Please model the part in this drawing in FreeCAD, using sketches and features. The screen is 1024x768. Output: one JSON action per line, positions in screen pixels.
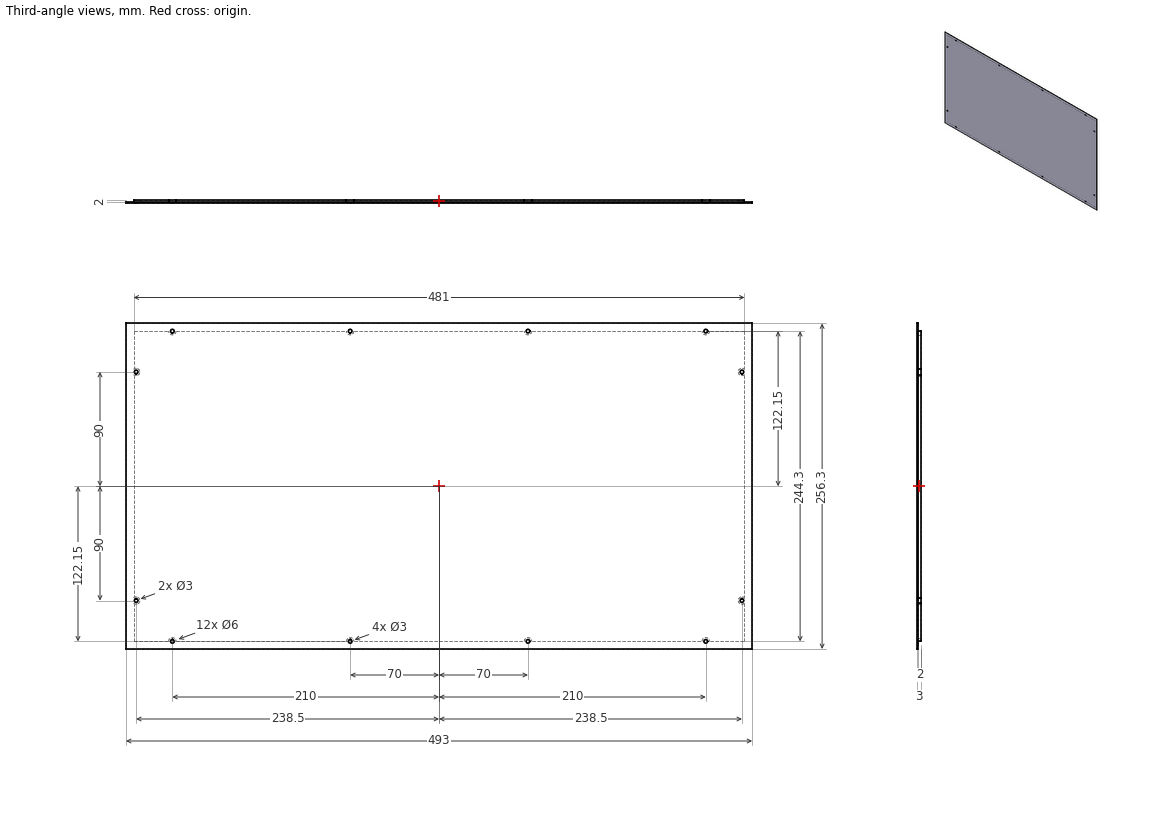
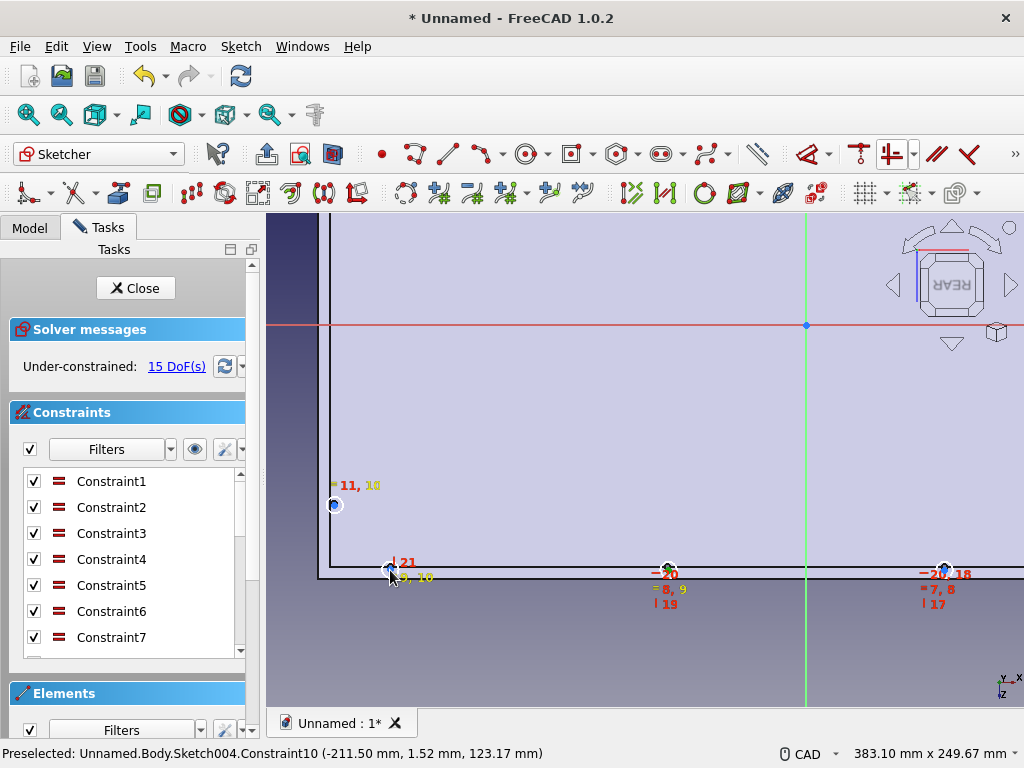
{"action": "scroll", "coordinate": [390, 570], "scroll_direction": "up", "scroll_amount": 4}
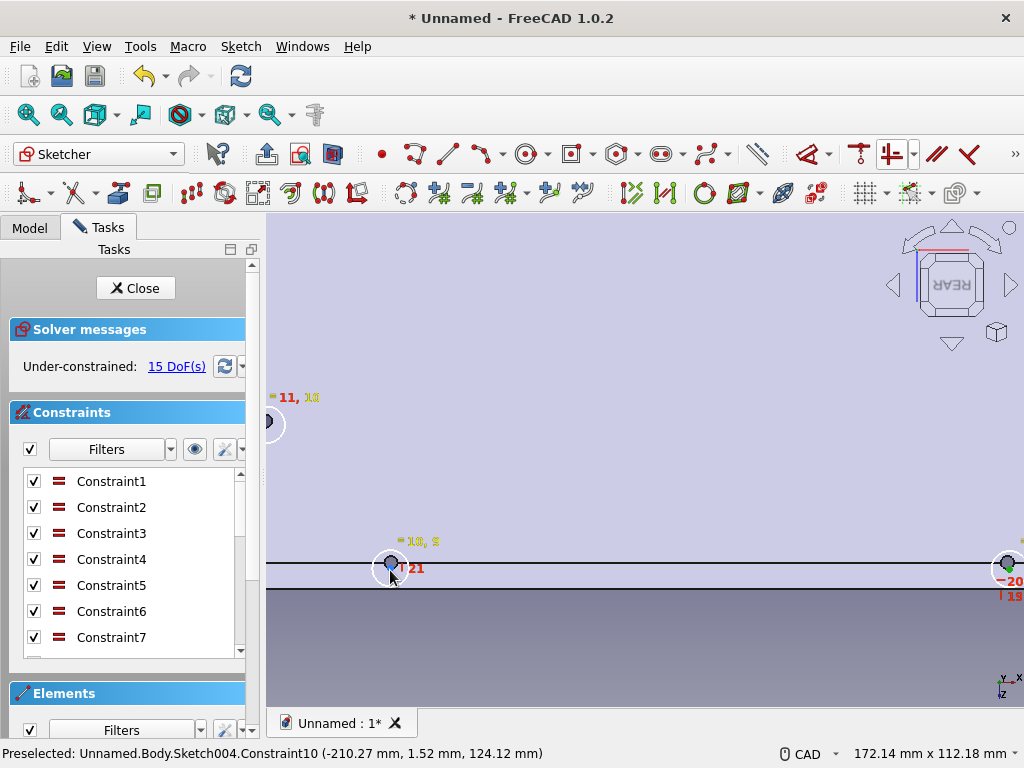
{"action": "left_click", "coordinate": [391, 568]}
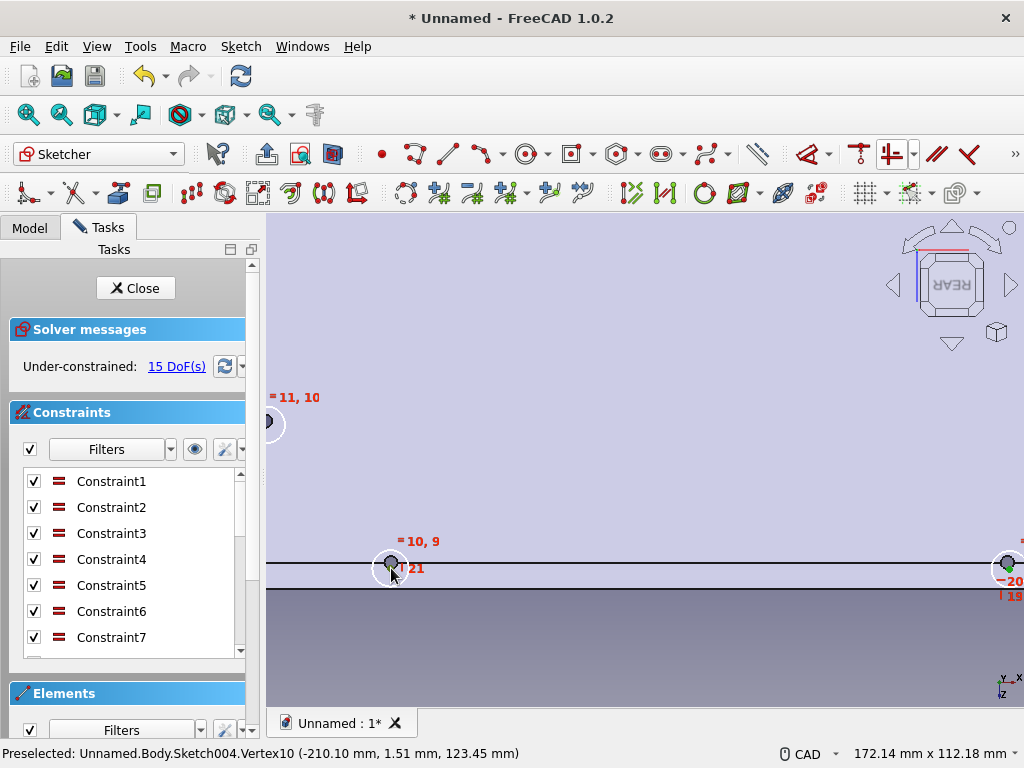
{"action": "left_click", "coordinate": [914, 154]}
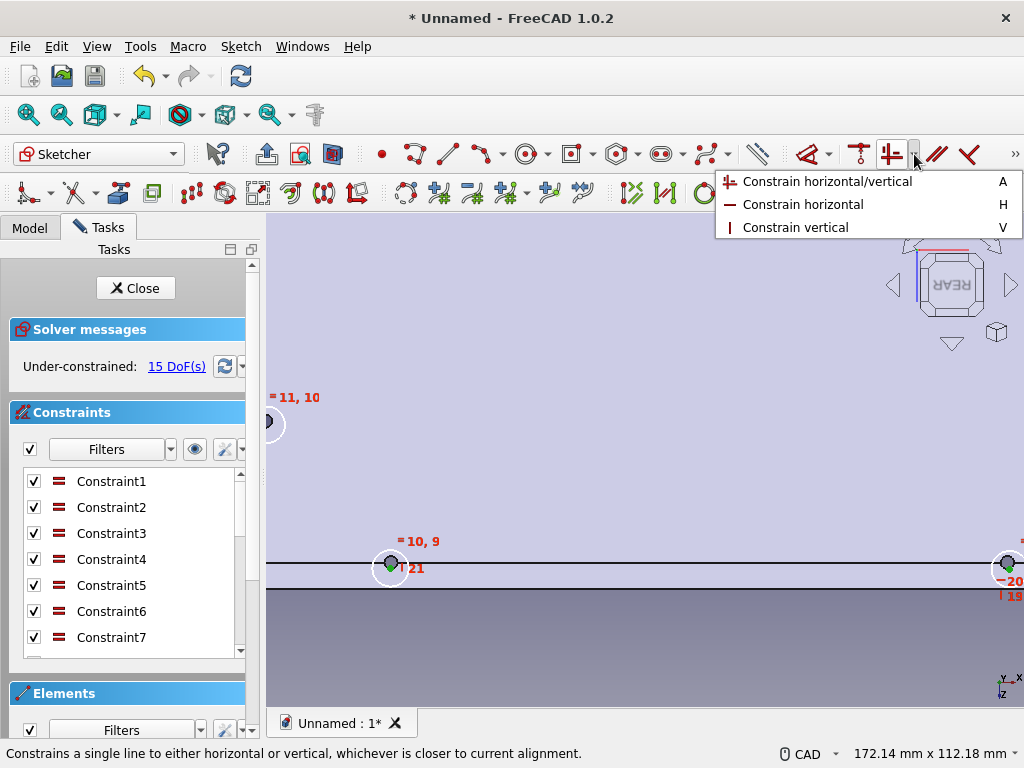
{"action": "left_click", "coordinate": [869, 204]}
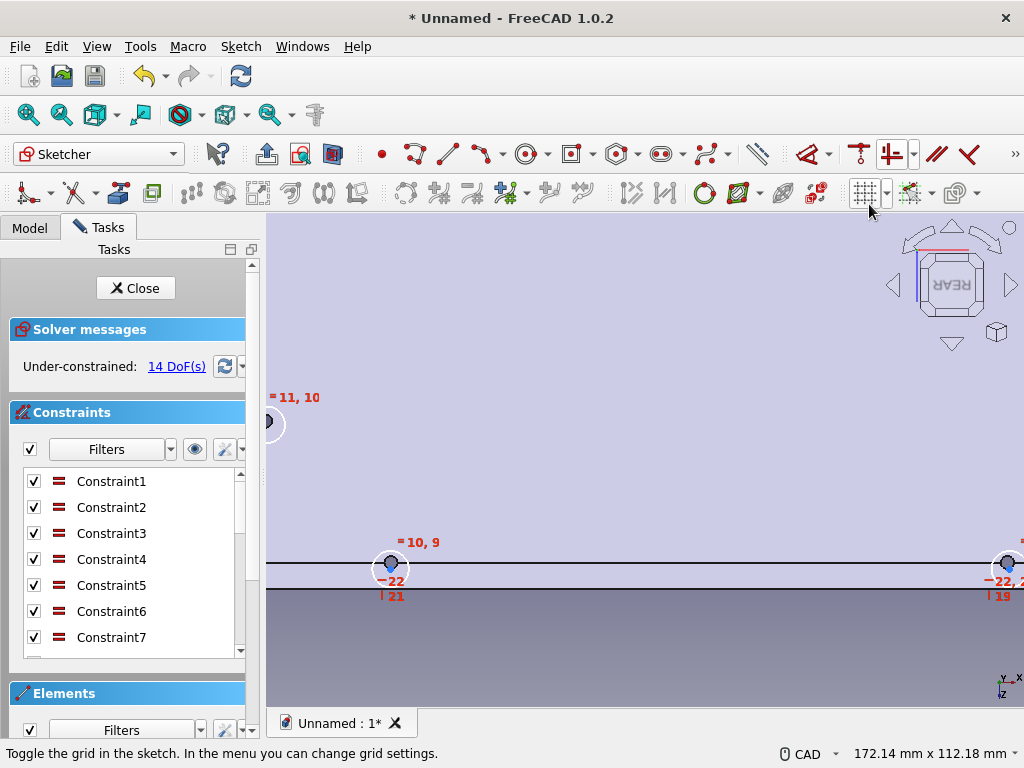
{"action": "scroll", "coordinate": [389, 570], "scroll_direction": "down", "scroll_amount": 8}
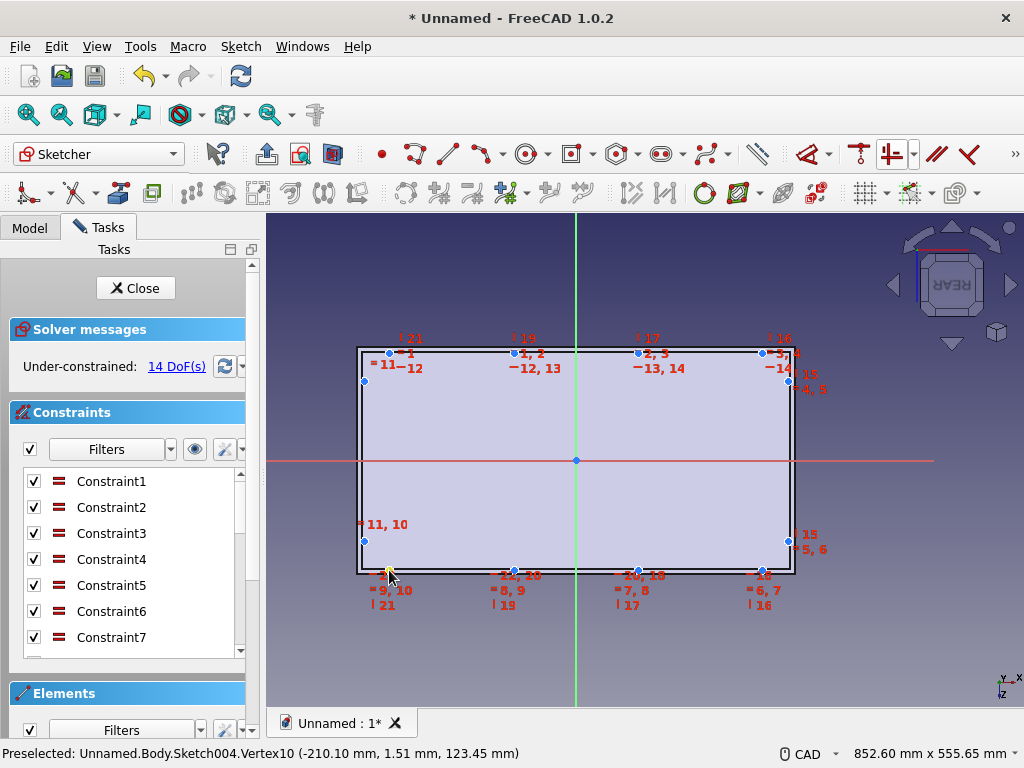
{"action": "left_click", "coordinate": [364, 541]}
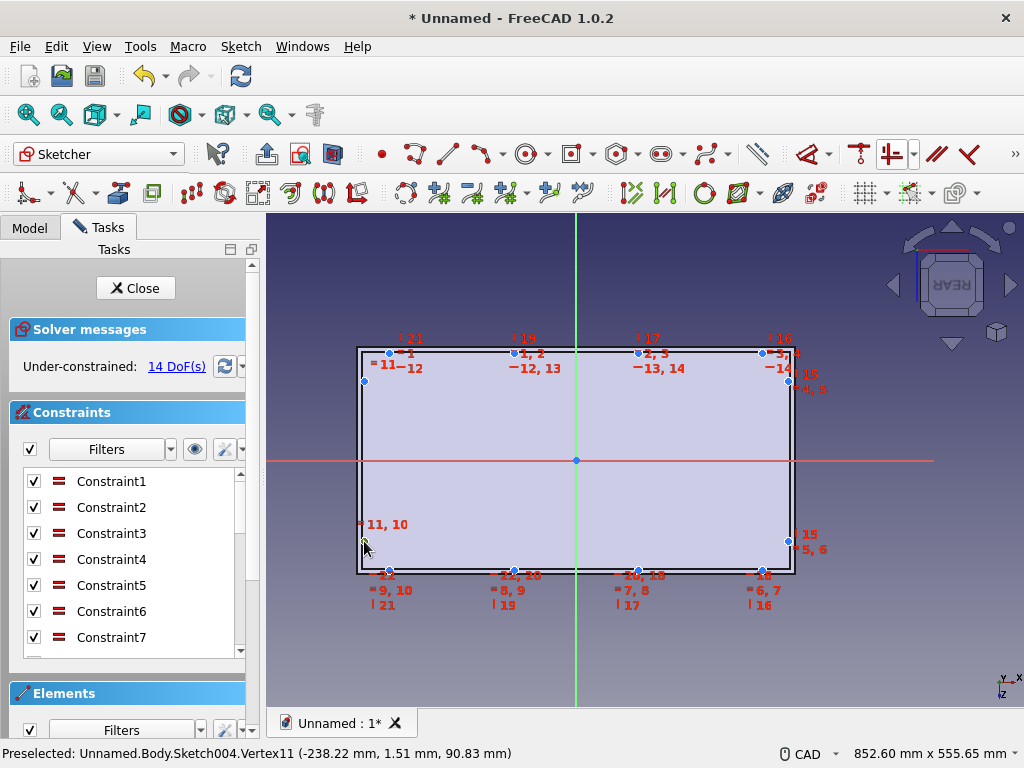
{"action": "left_click", "coordinate": [364, 381]}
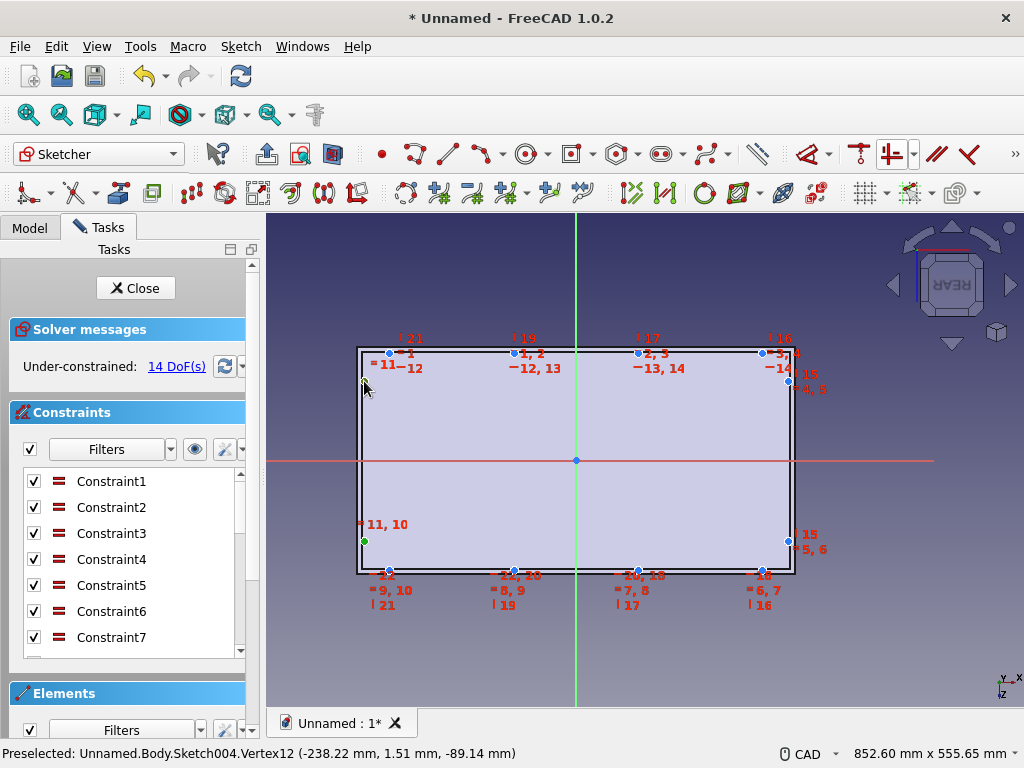
{"action": "left_click", "coordinate": [914, 154]}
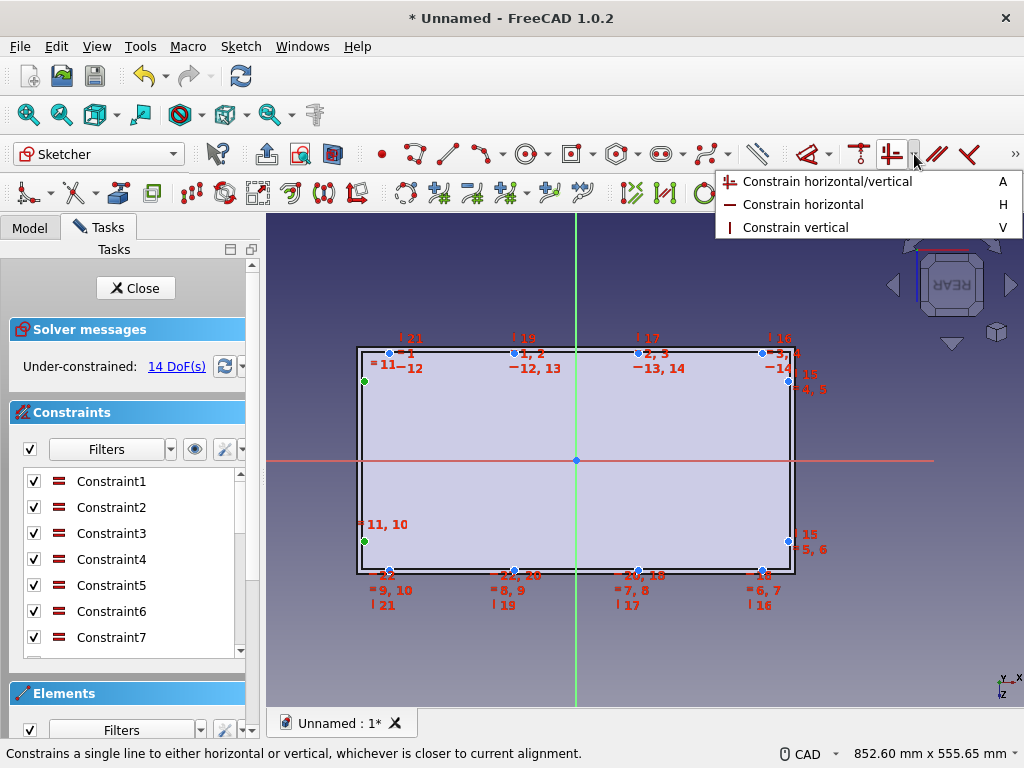
{"action": "left_click", "coordinate": [869, 228]}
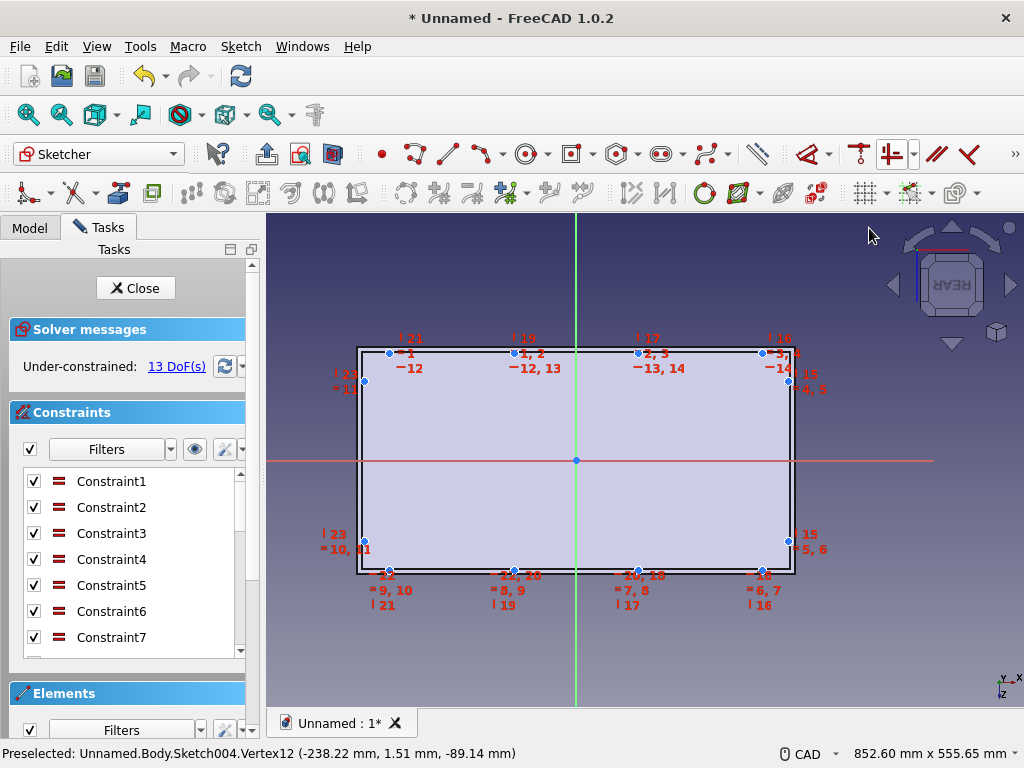
{"action": "left_click", "coordinate": [806, 154]}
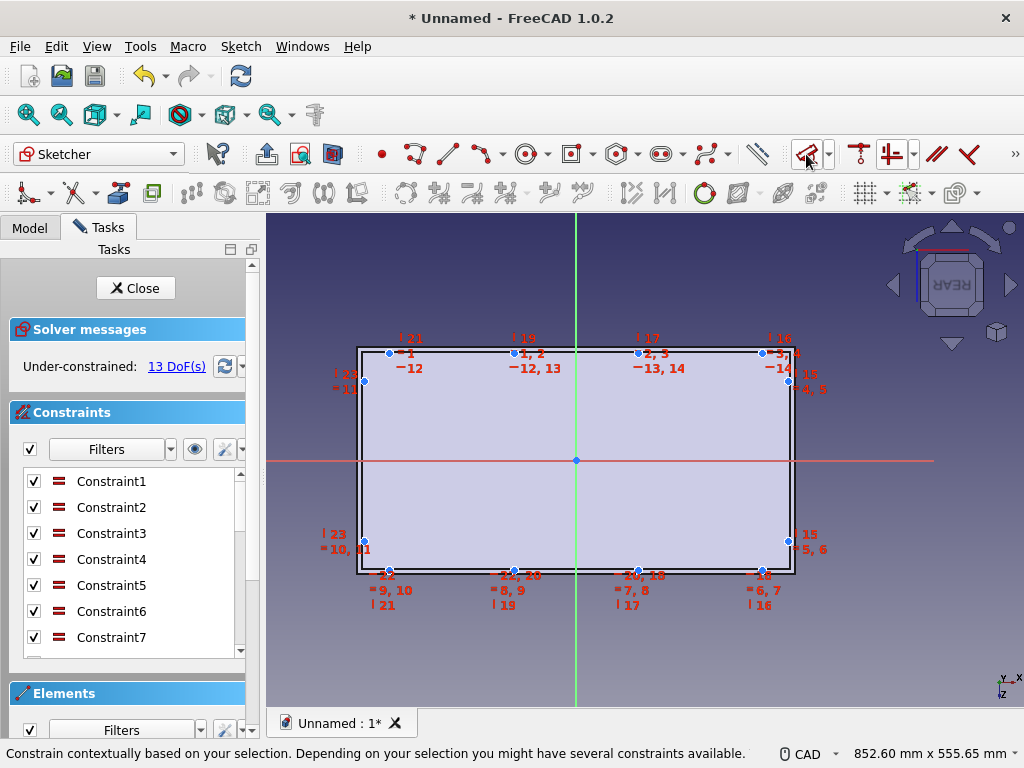
{"action": "scroll", "coordinate": [390, 350], "scroll_direction": "up", "scroll_amount": 11}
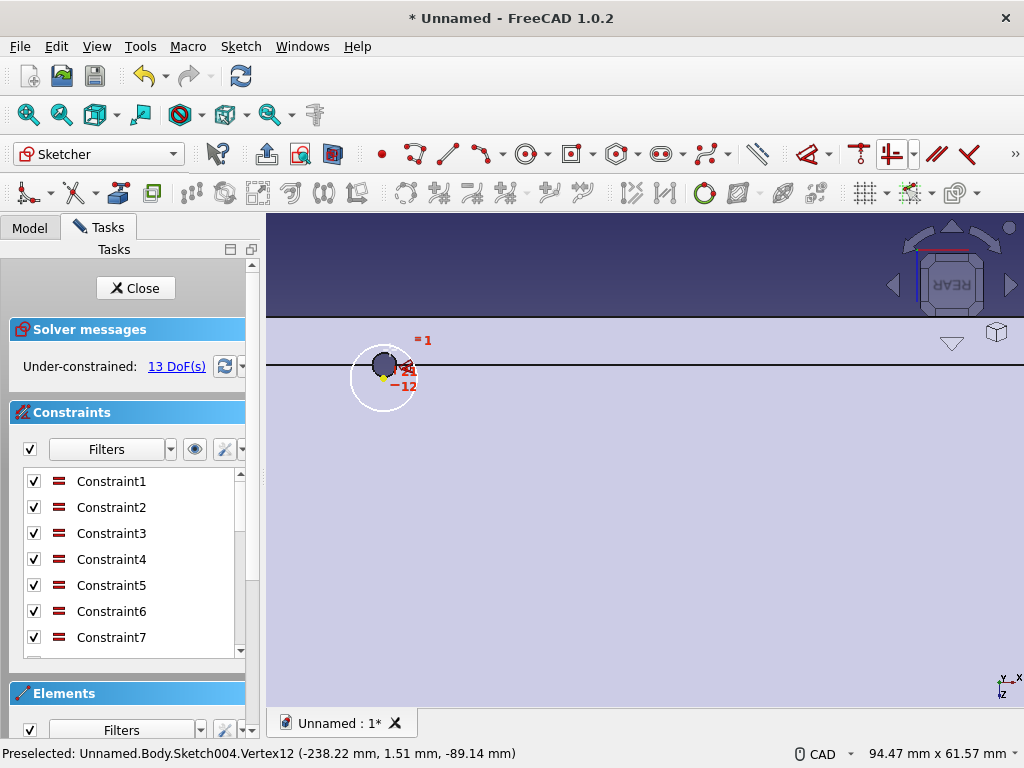
{"action": "left_click", "coordinate": [385, 345]}
{"action": "left_click", "coordinate": [386, 313]}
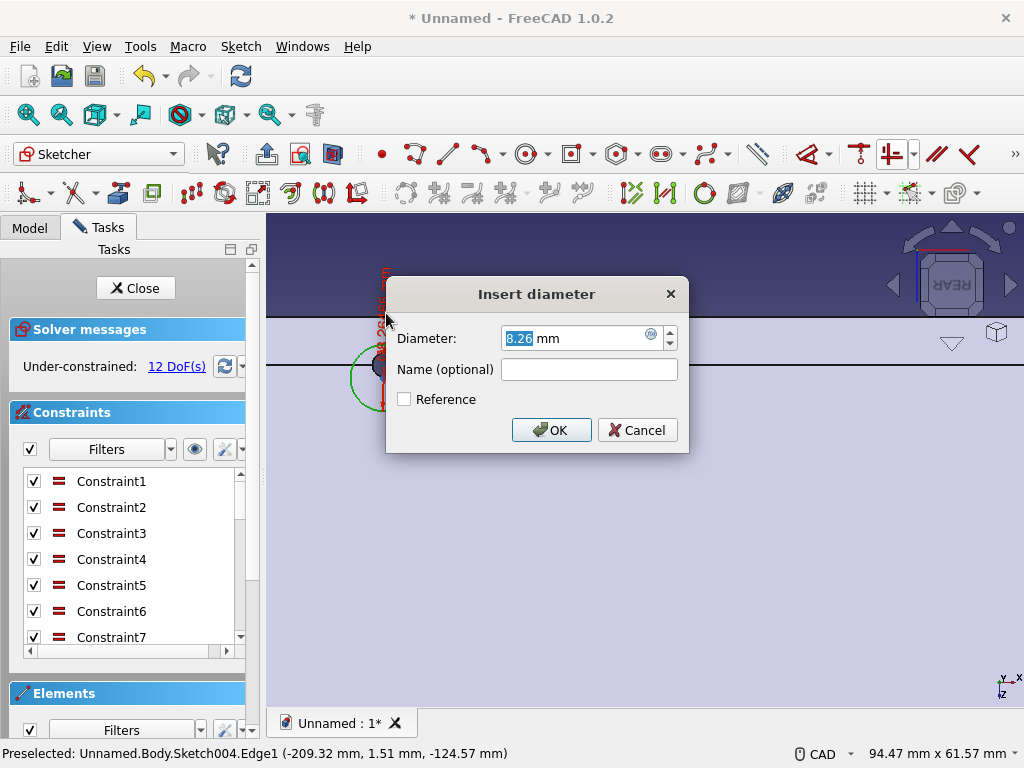
{"action": "type", "text": "6"}
{"action": "key", "text": "Return"}